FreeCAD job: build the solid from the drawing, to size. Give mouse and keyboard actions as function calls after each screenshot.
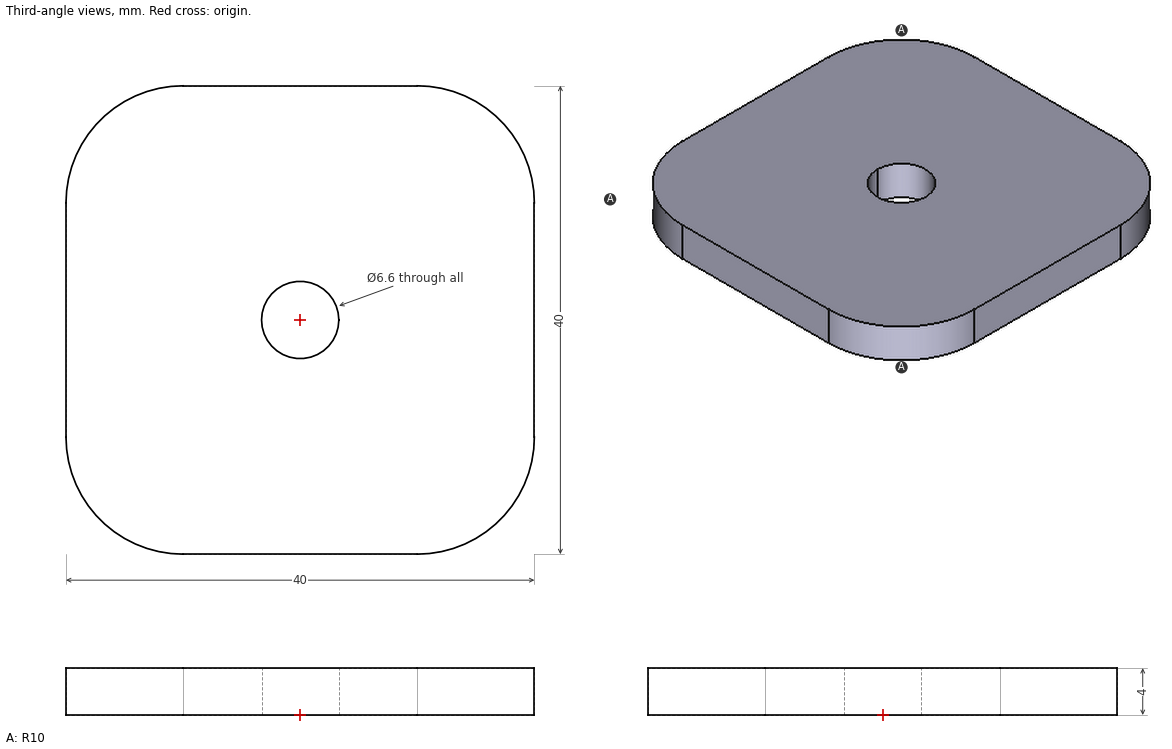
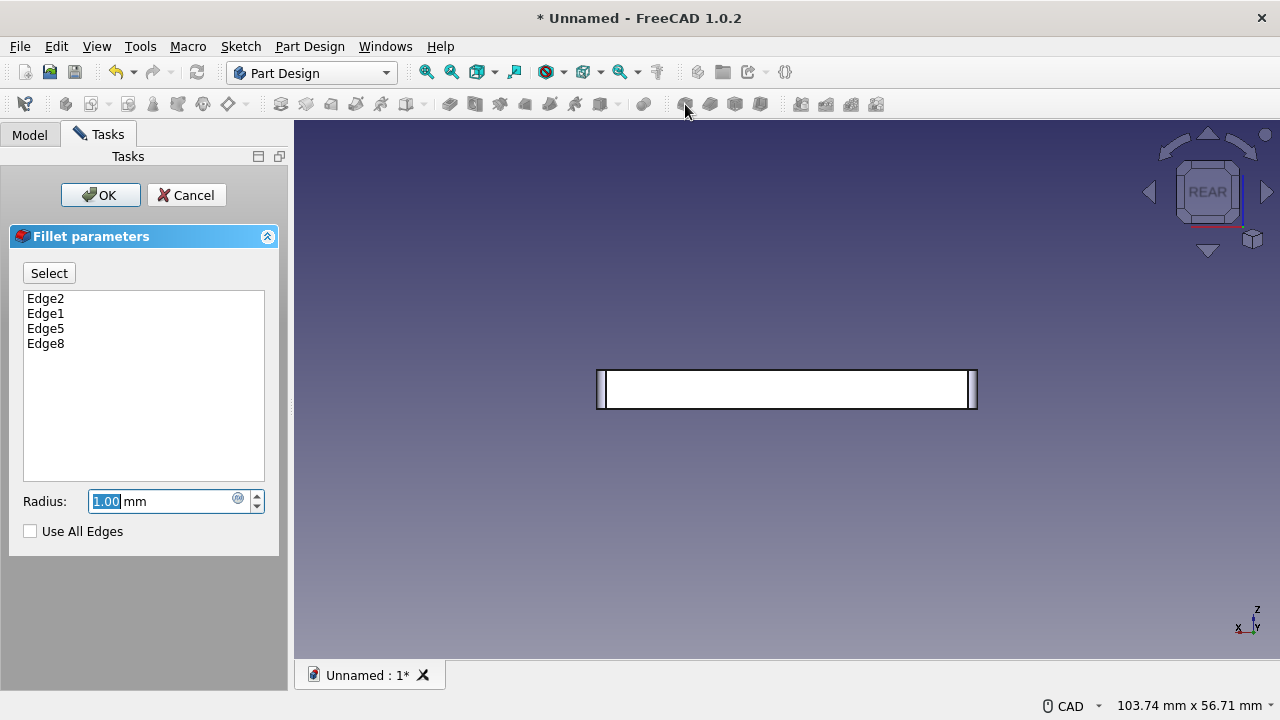
text(10)
key(Tab)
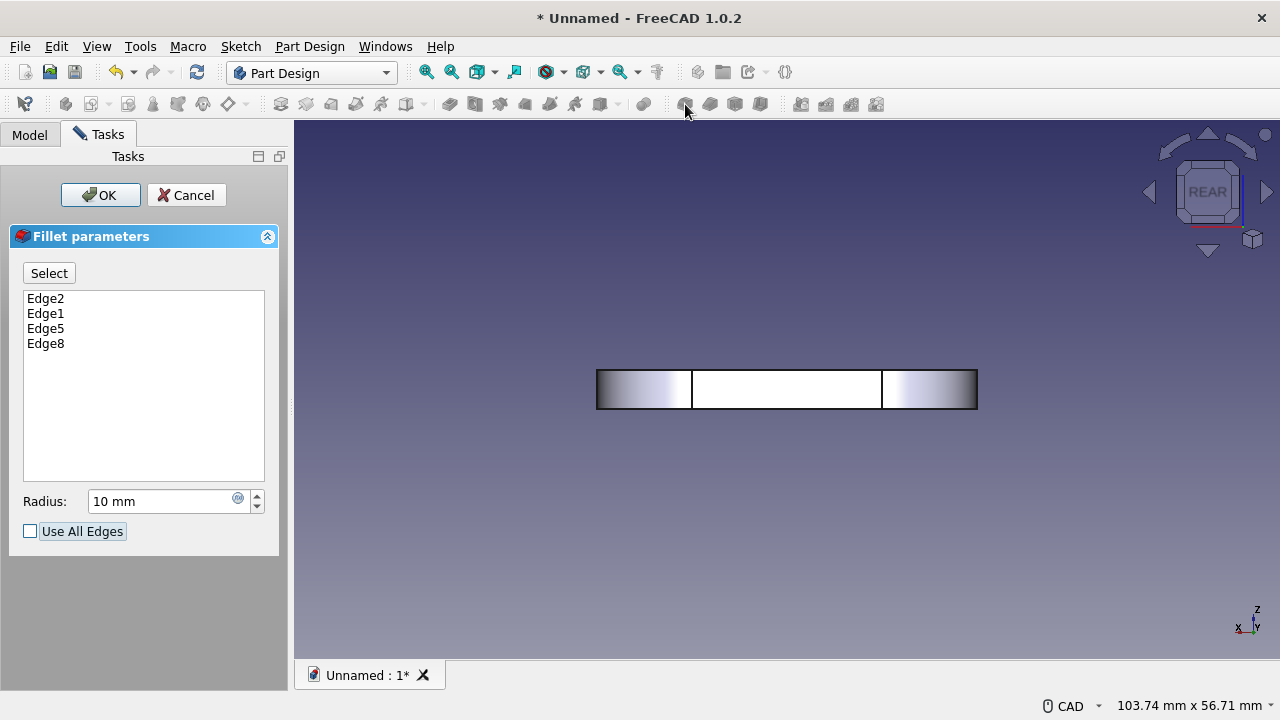
click(101, 195)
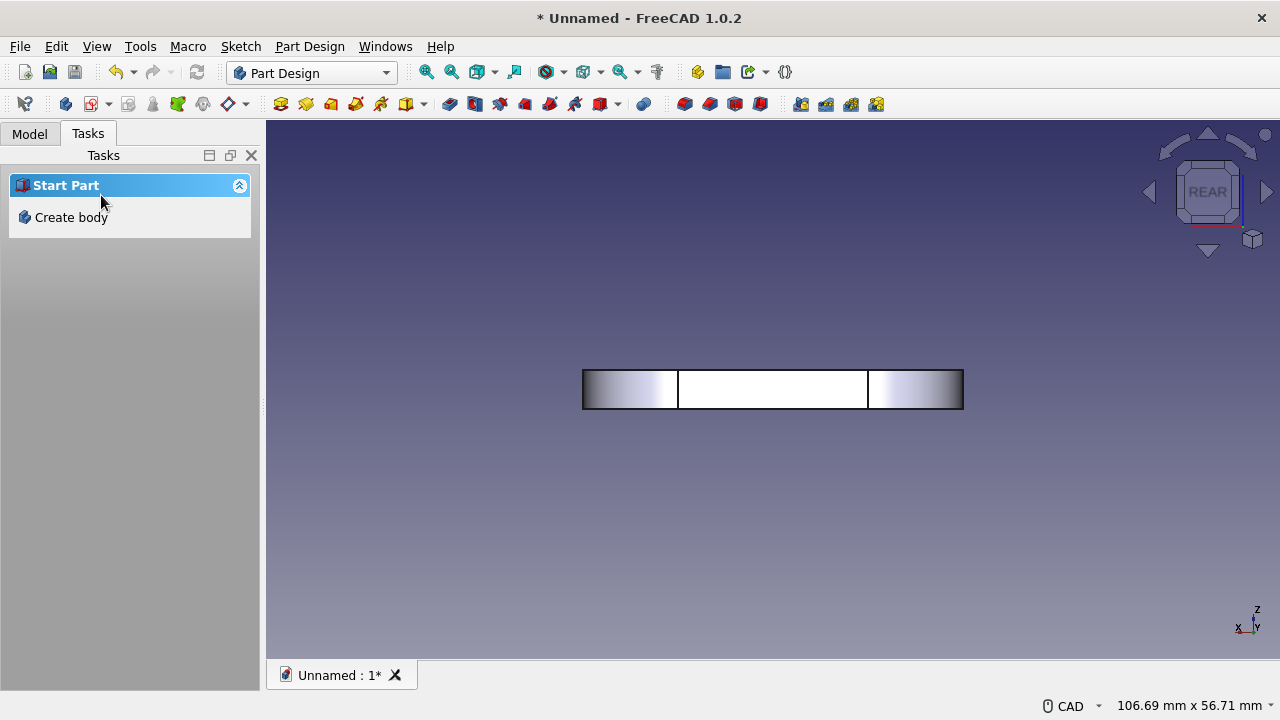
click(427, 72)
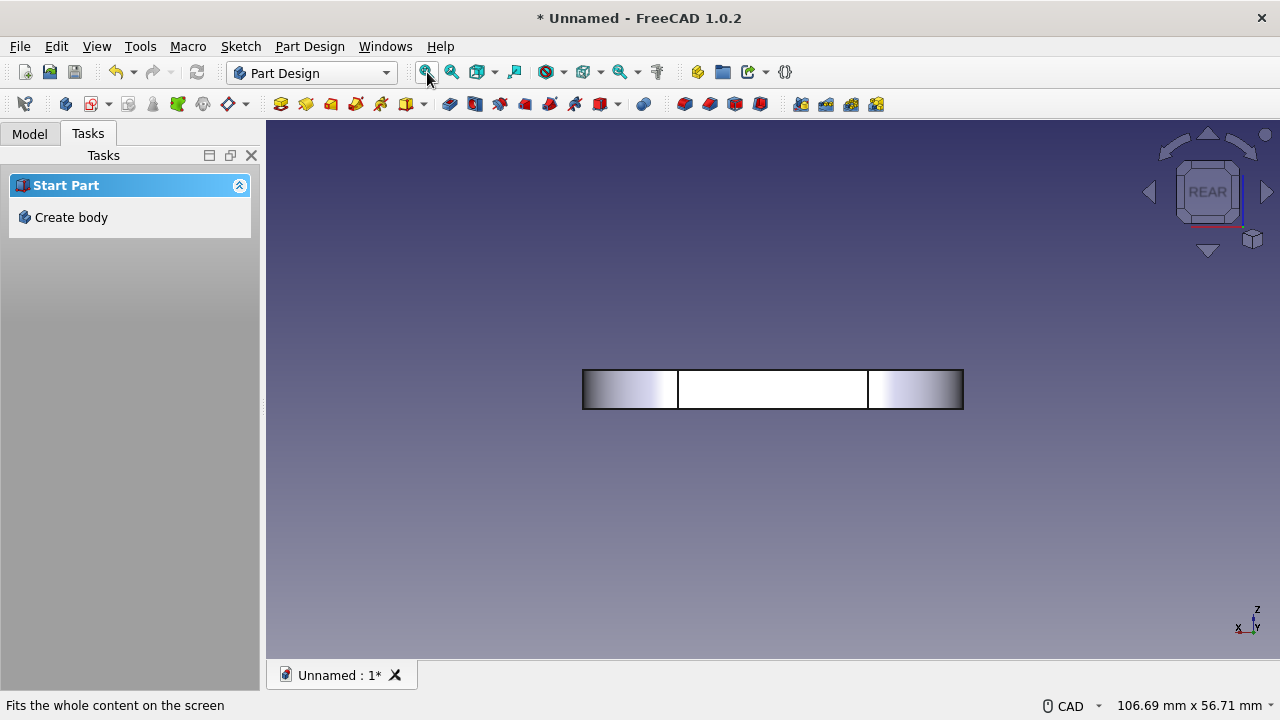
click(90, 104)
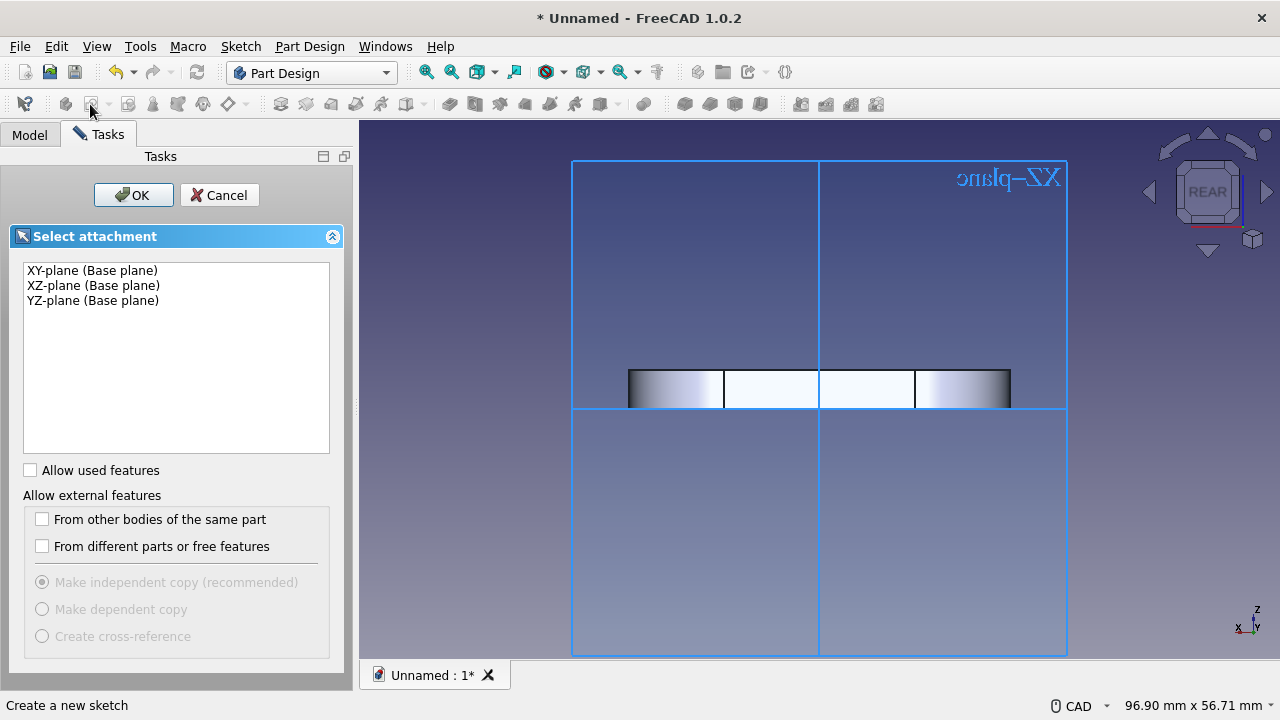
click(84, 270)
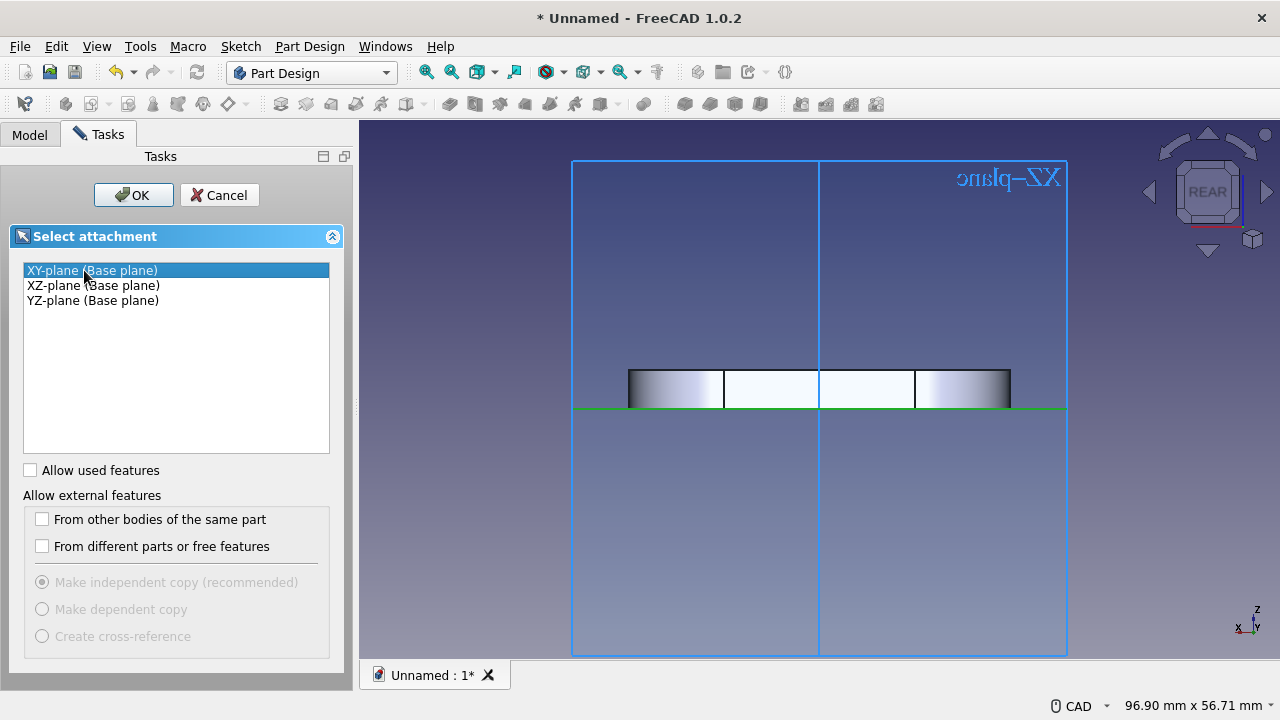
click(134, 195)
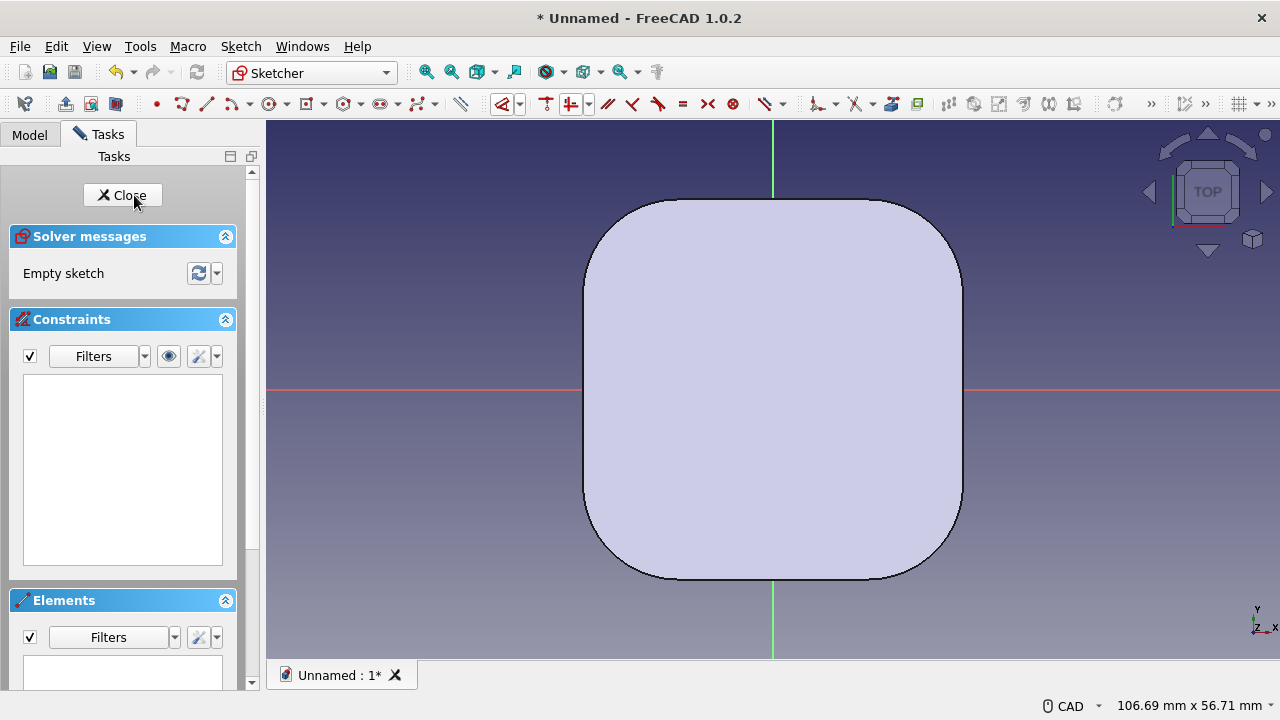
click(116, 104)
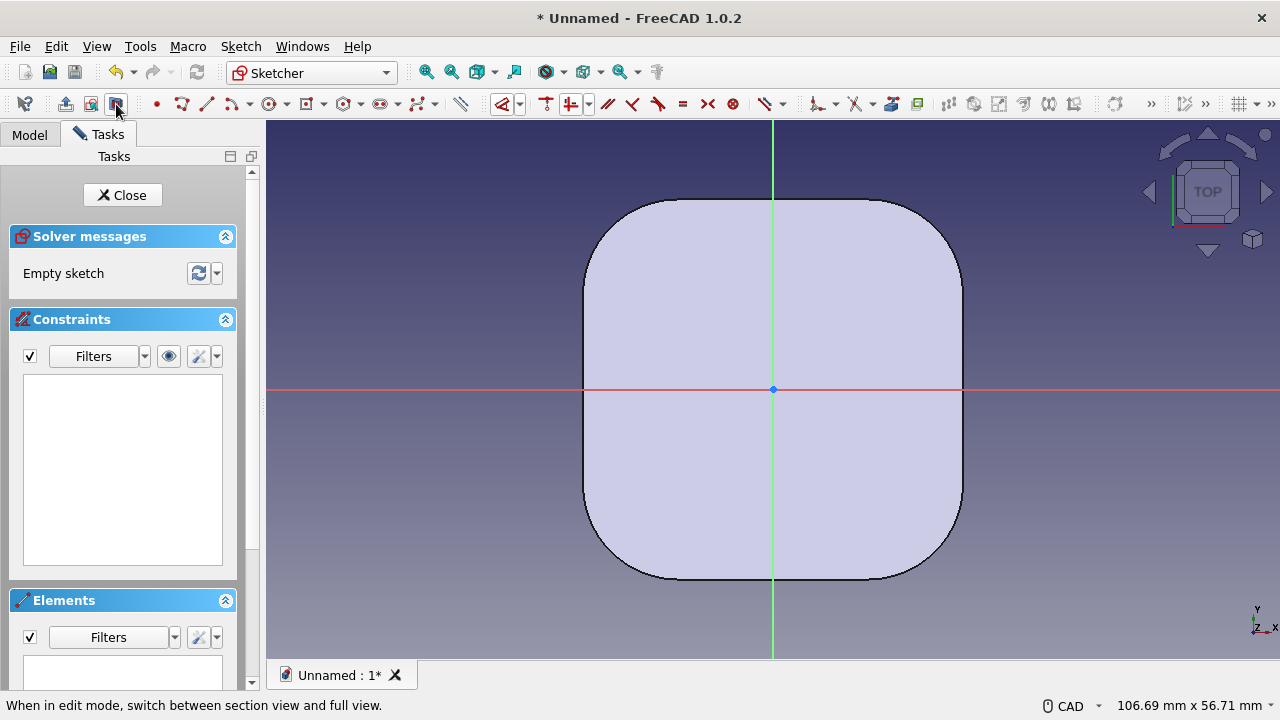
scroll(790, 390, up, 8)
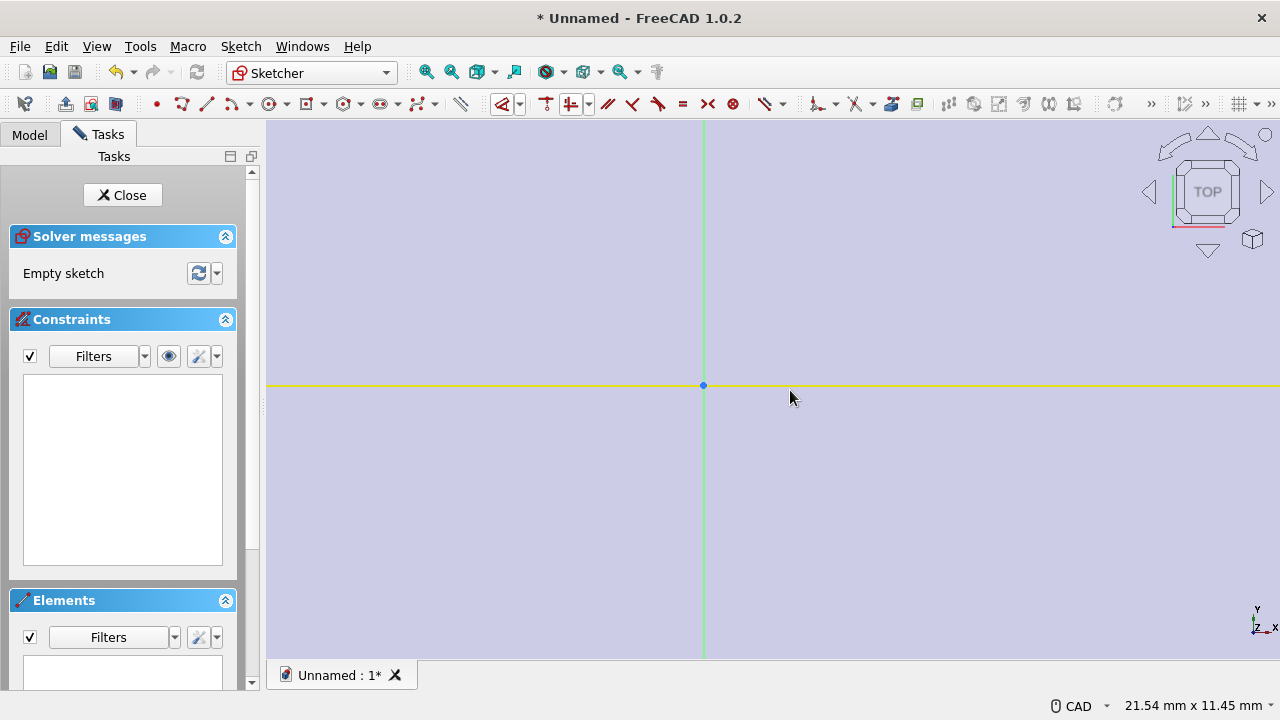
click(268, 104)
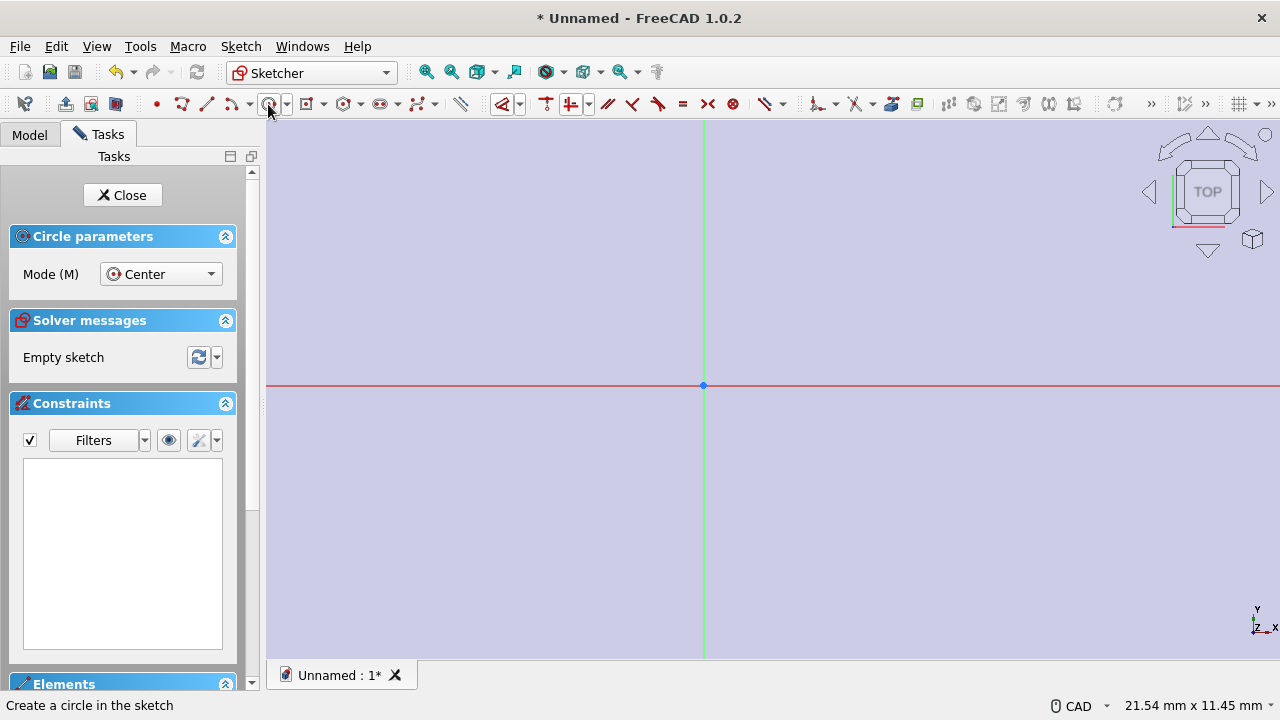
click(704, 386)
click(814, 276)
key(Escape)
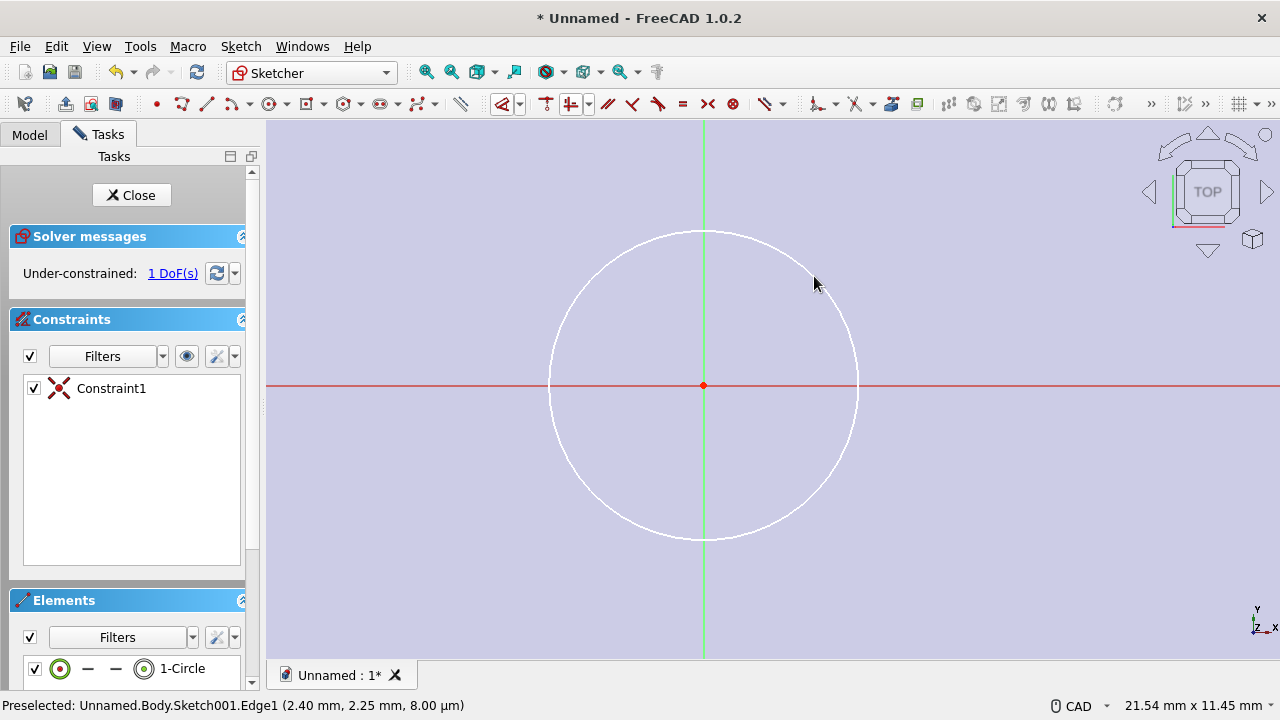
click(813, 276)